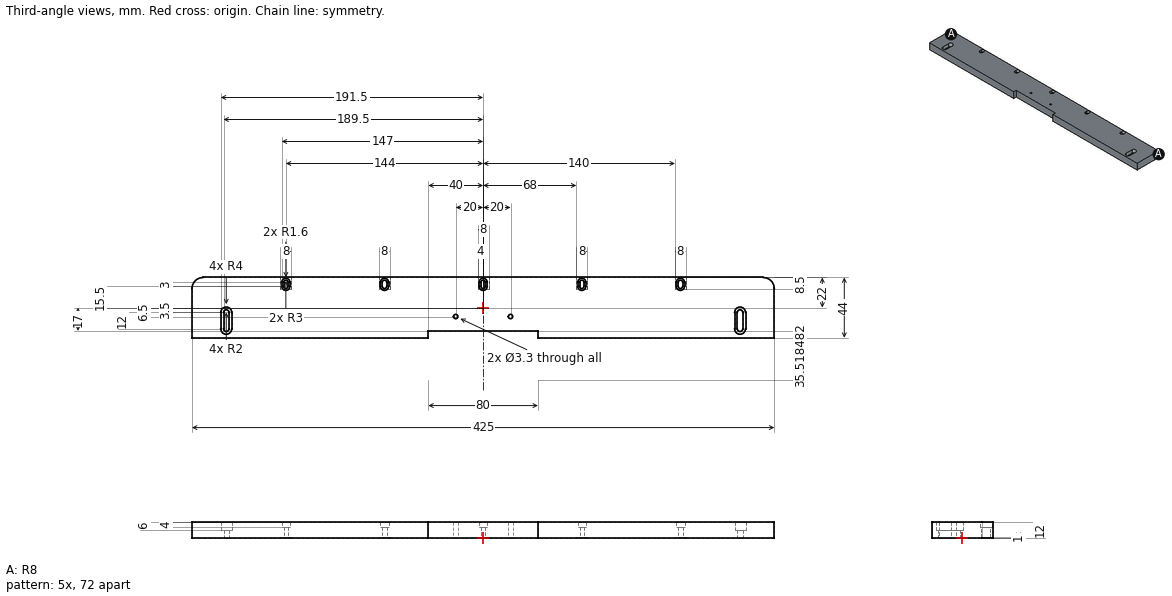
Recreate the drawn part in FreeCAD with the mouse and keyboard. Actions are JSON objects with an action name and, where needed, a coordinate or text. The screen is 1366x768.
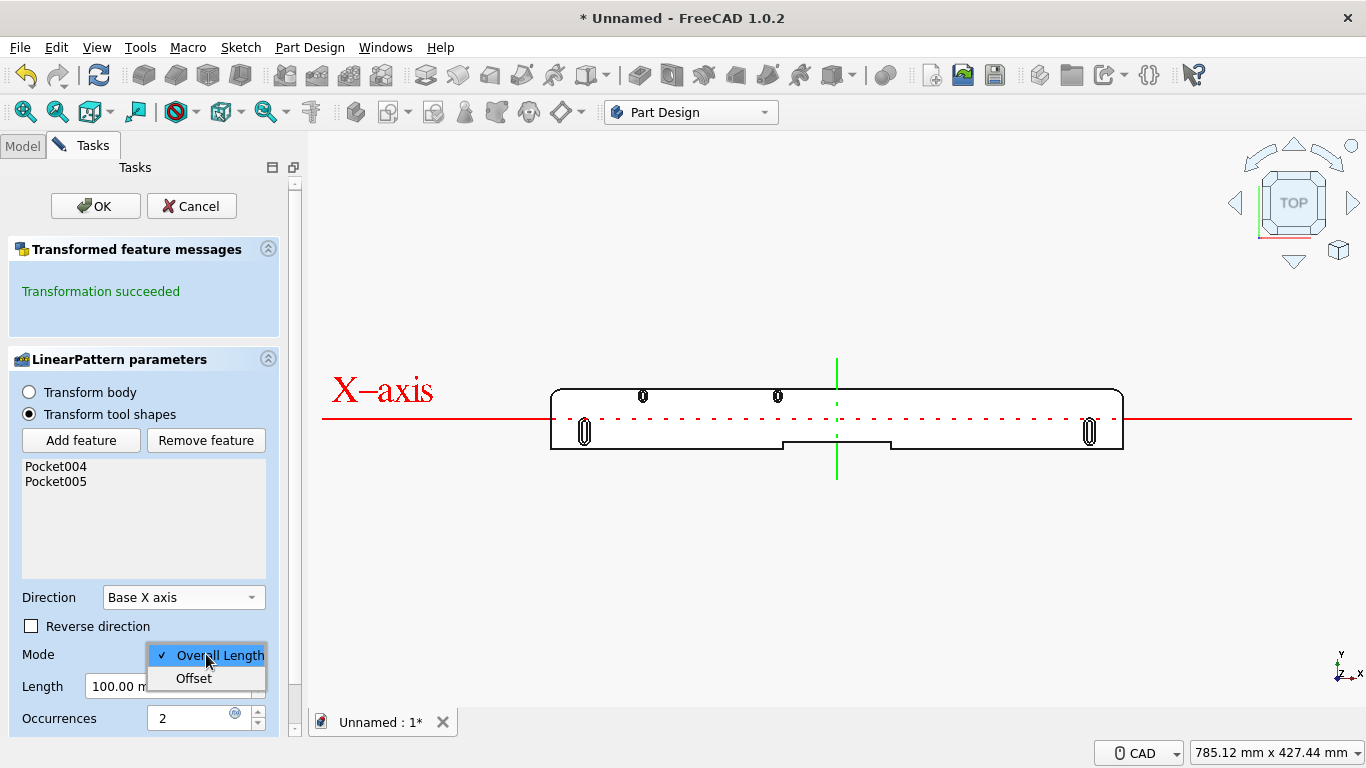
{"action": "left_click", "coordinate": [206, 678]}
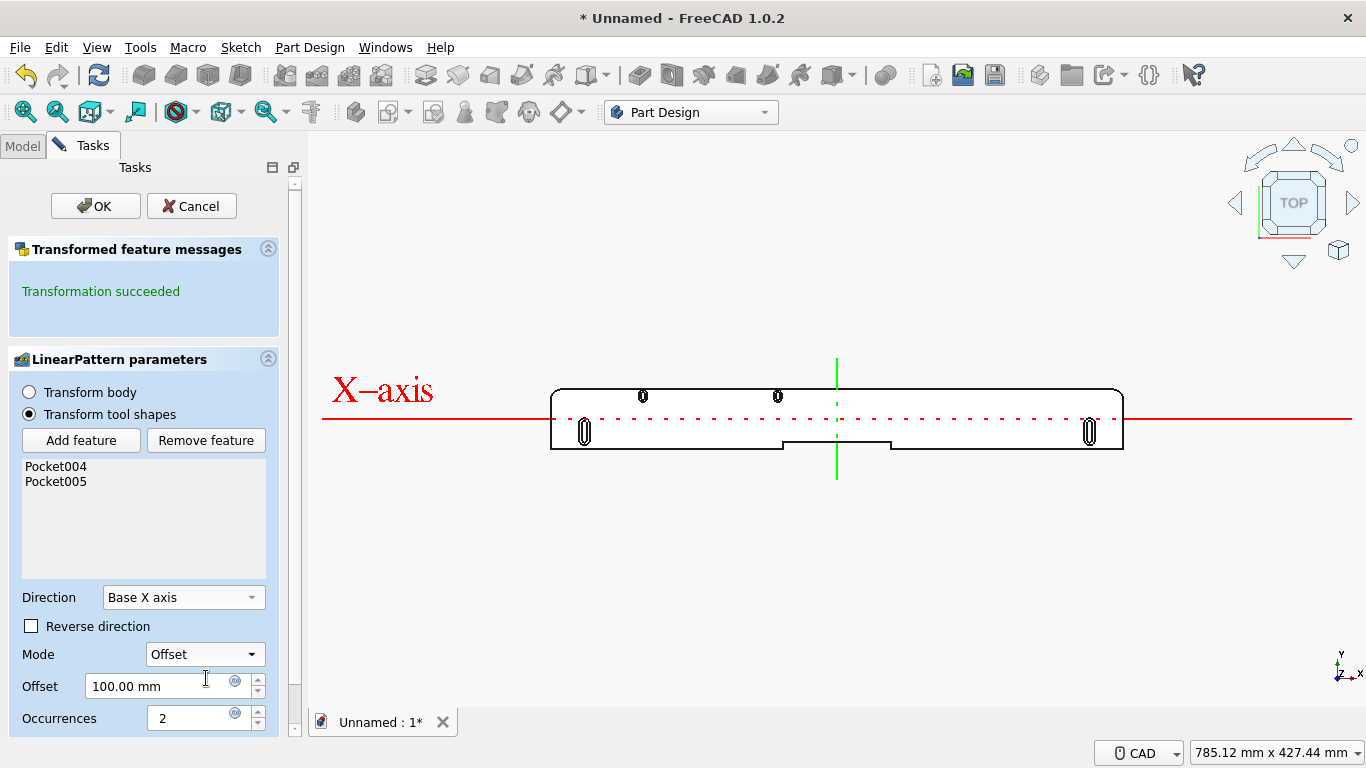
{"action": "triple_click", "coordinate": [168, 686]}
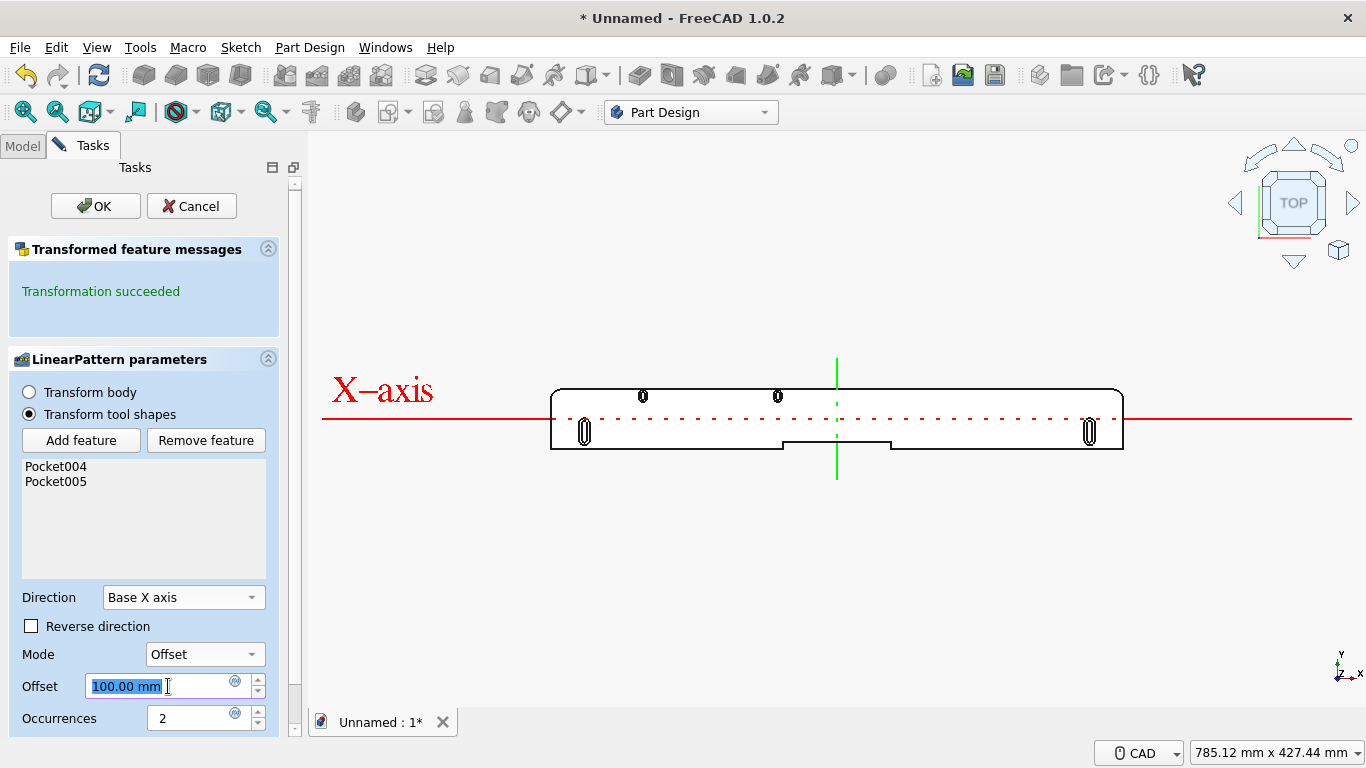
{"action": "type", "text": "72"}
{"action": "key", "text": "Tab"}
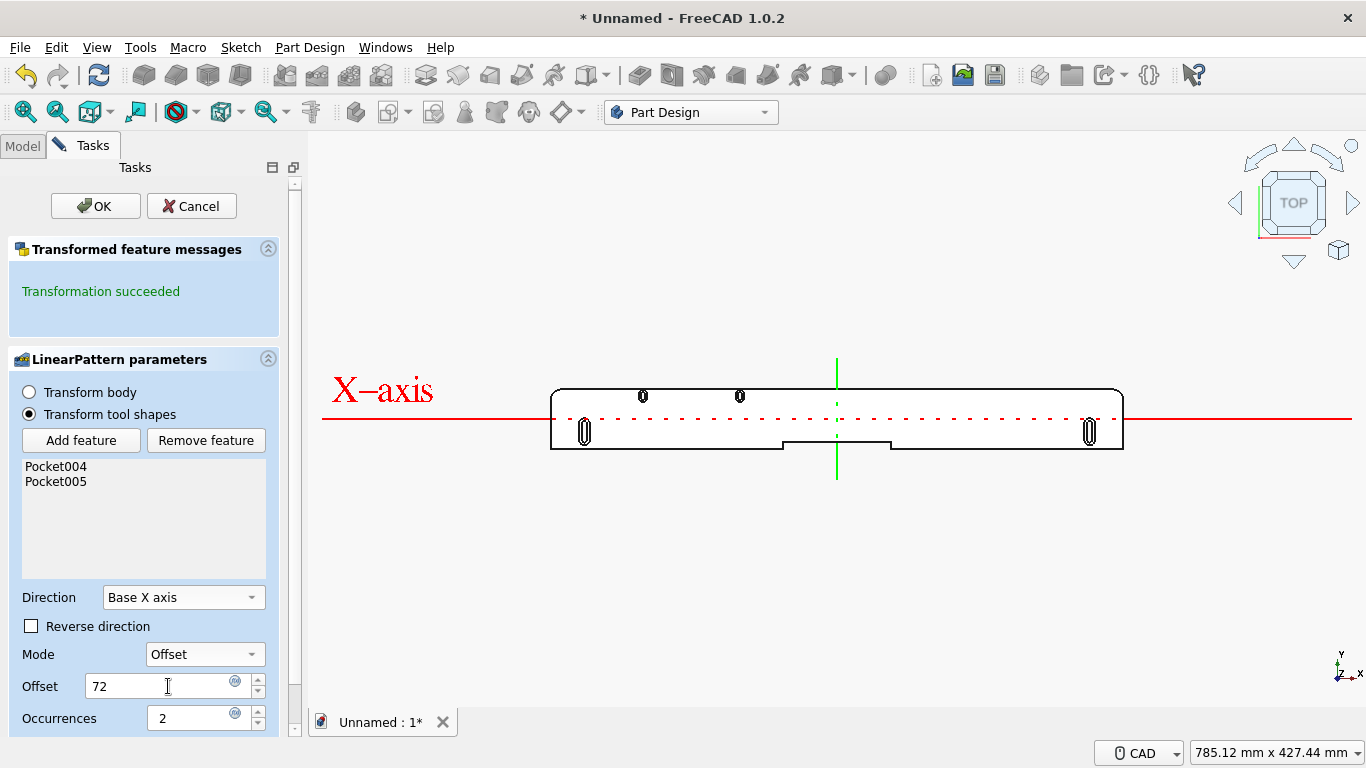
{"action": "triple_click", "coordinate": [198, 718]}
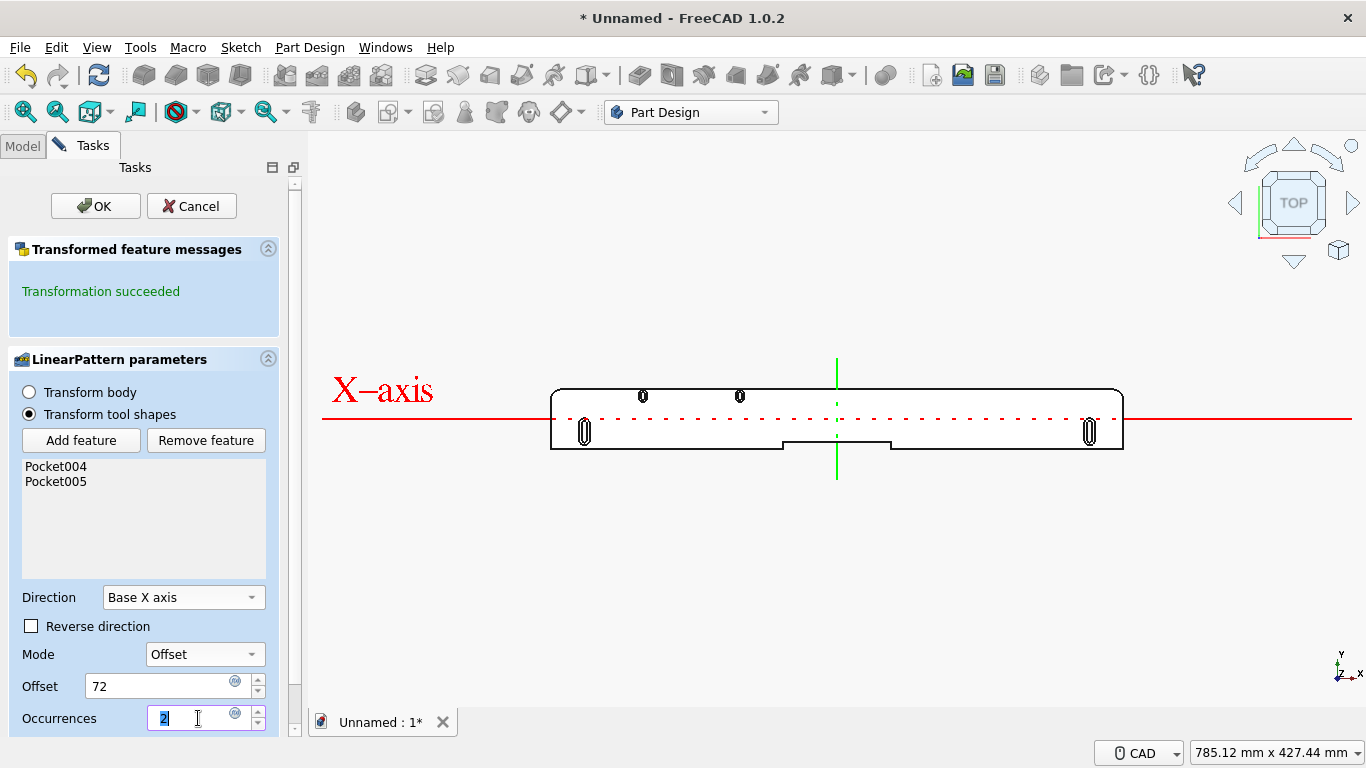
{"action": "type", "text": "5"}
{"action": "key", "text": "Tab"}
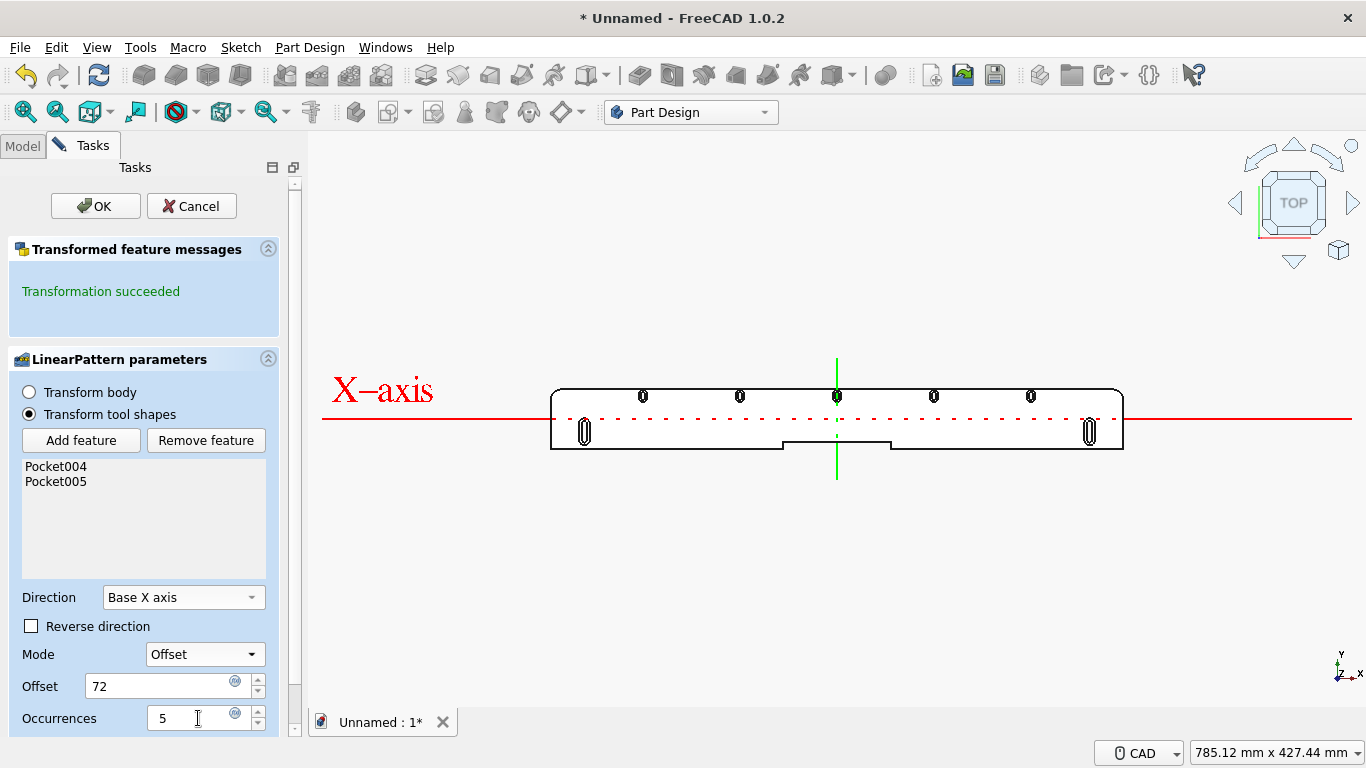
{"action": "left_click", "coordinate": [96, 206]}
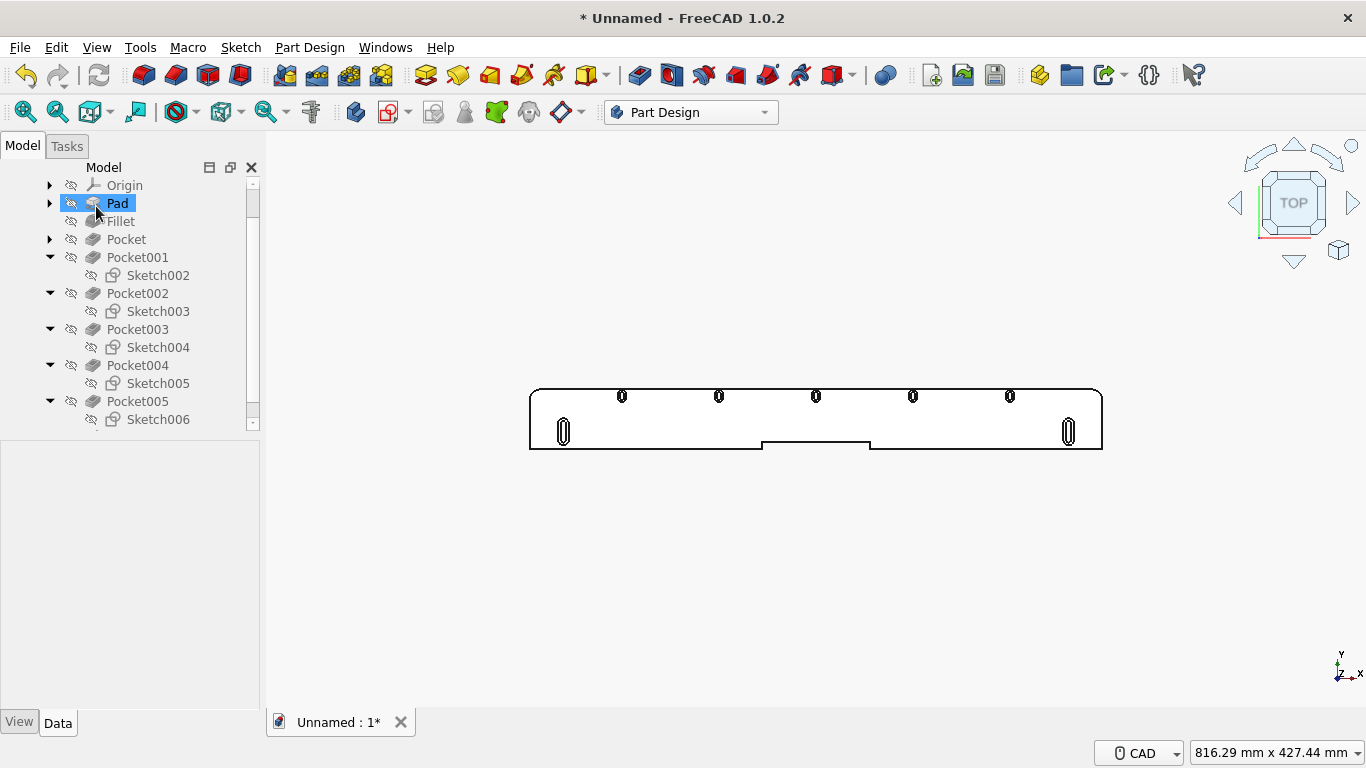
{"action": "left_click", "coordinate": [980, 418]}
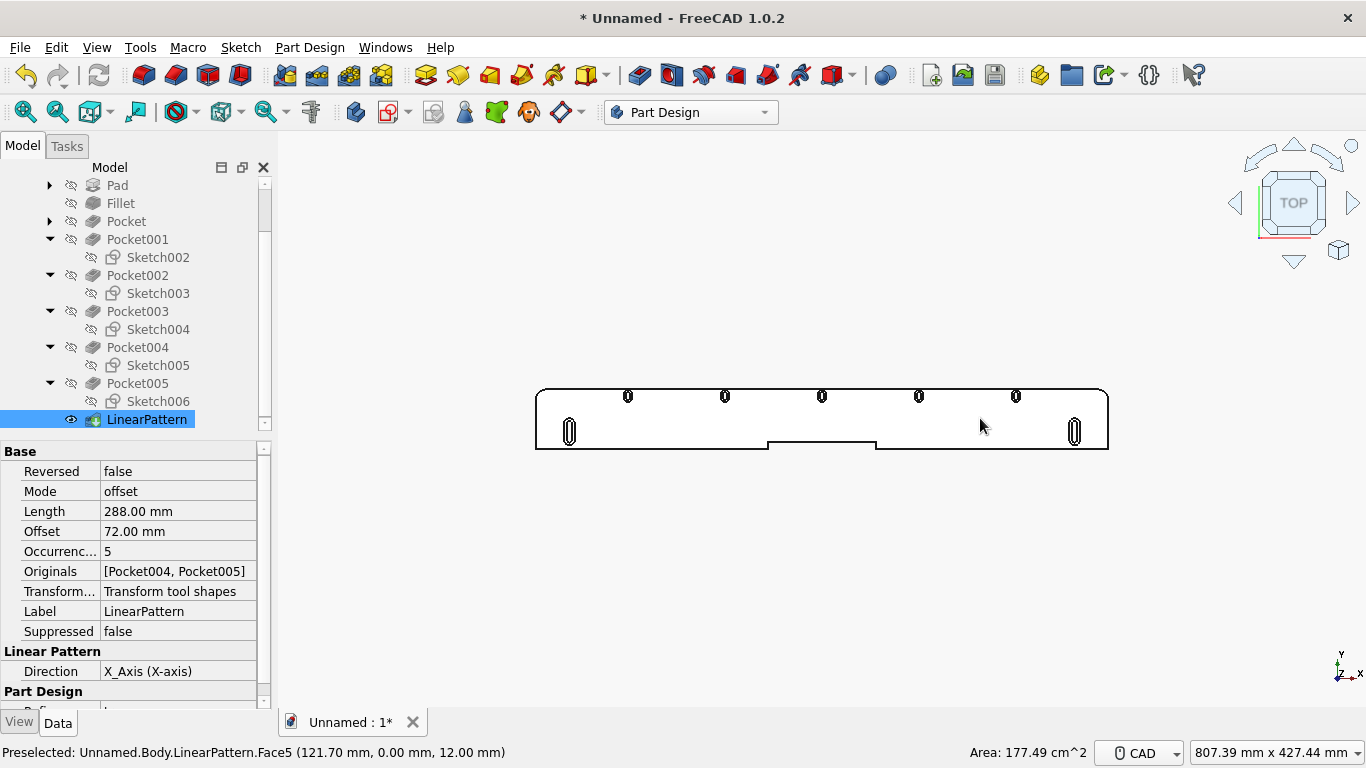
{"action": "left_click", "coordinate": [388, 112]}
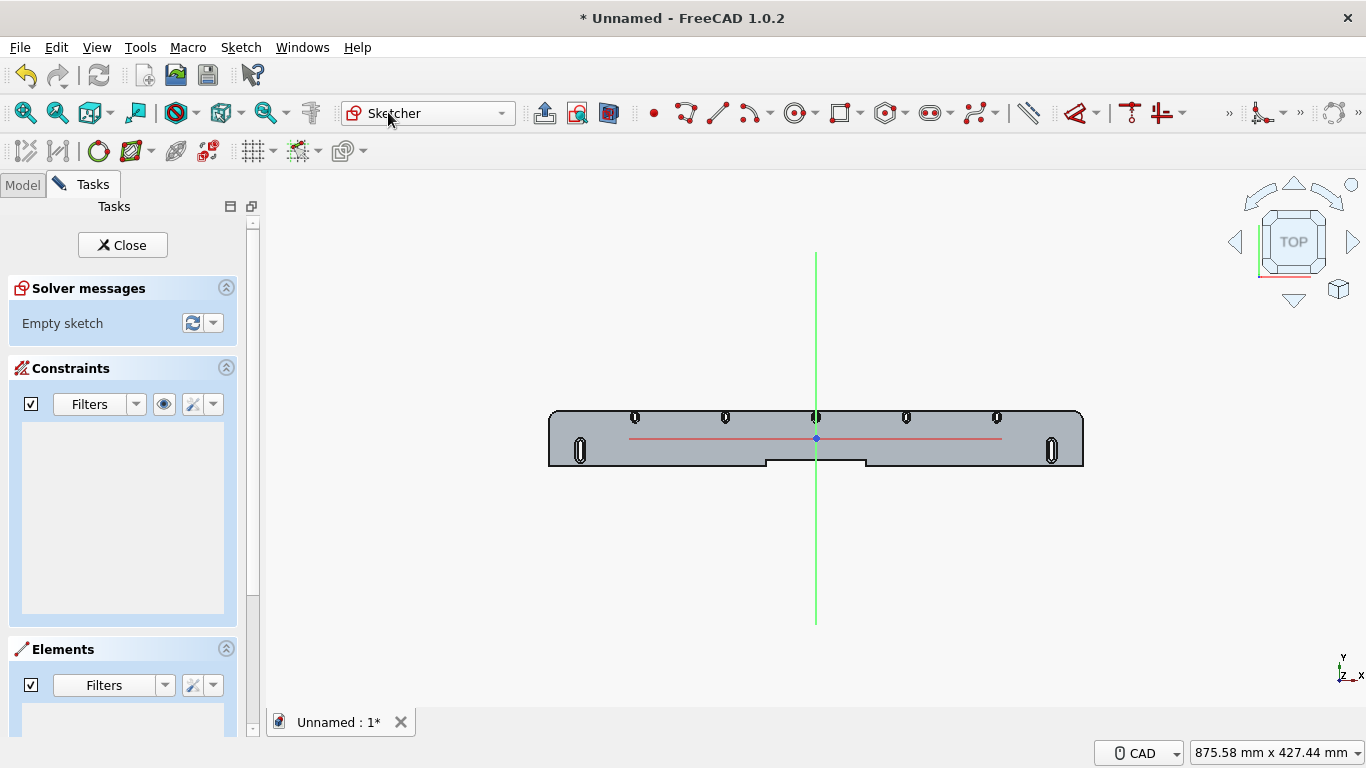
{"action": "scroll", "coordinate": [823, 444], "scroll_direction": "up", "scroll_amount": 12}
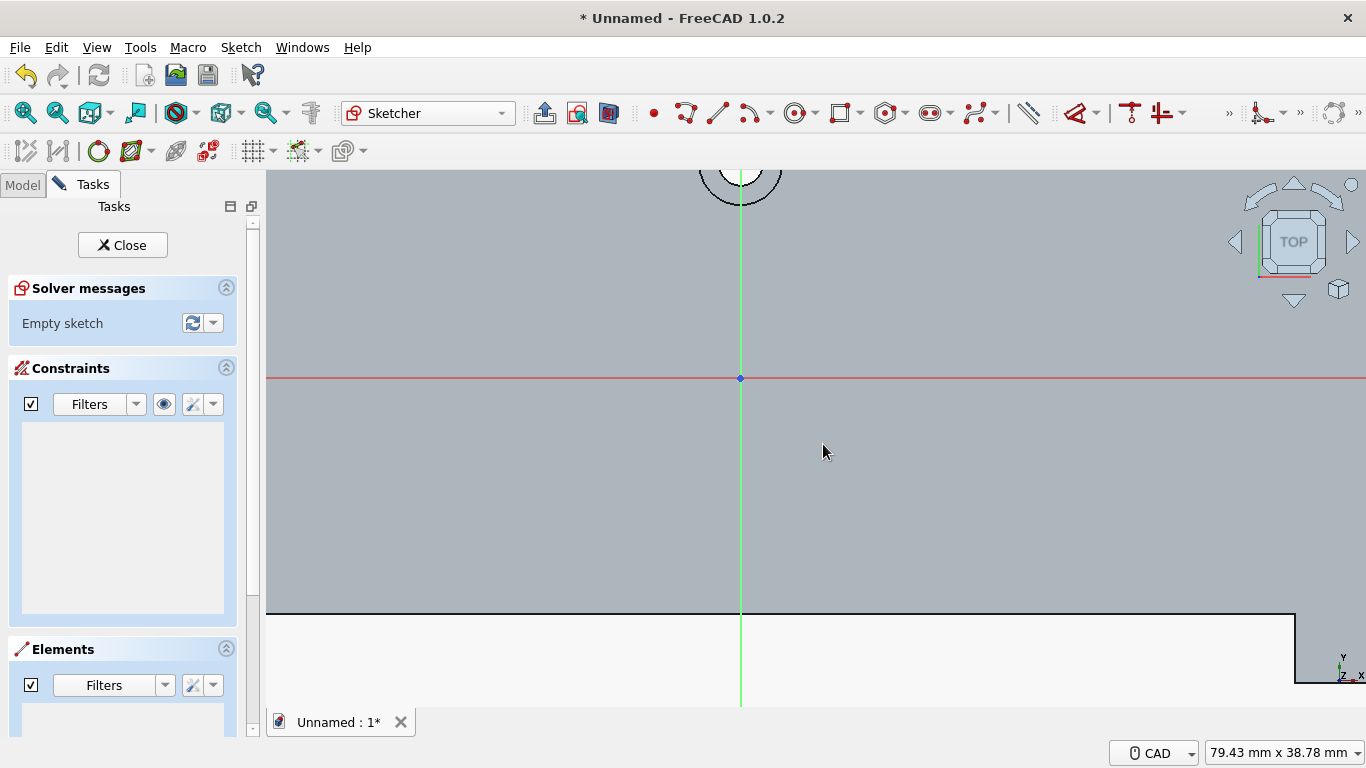
{"action": "left_click", "coordinate": [796, 114]}